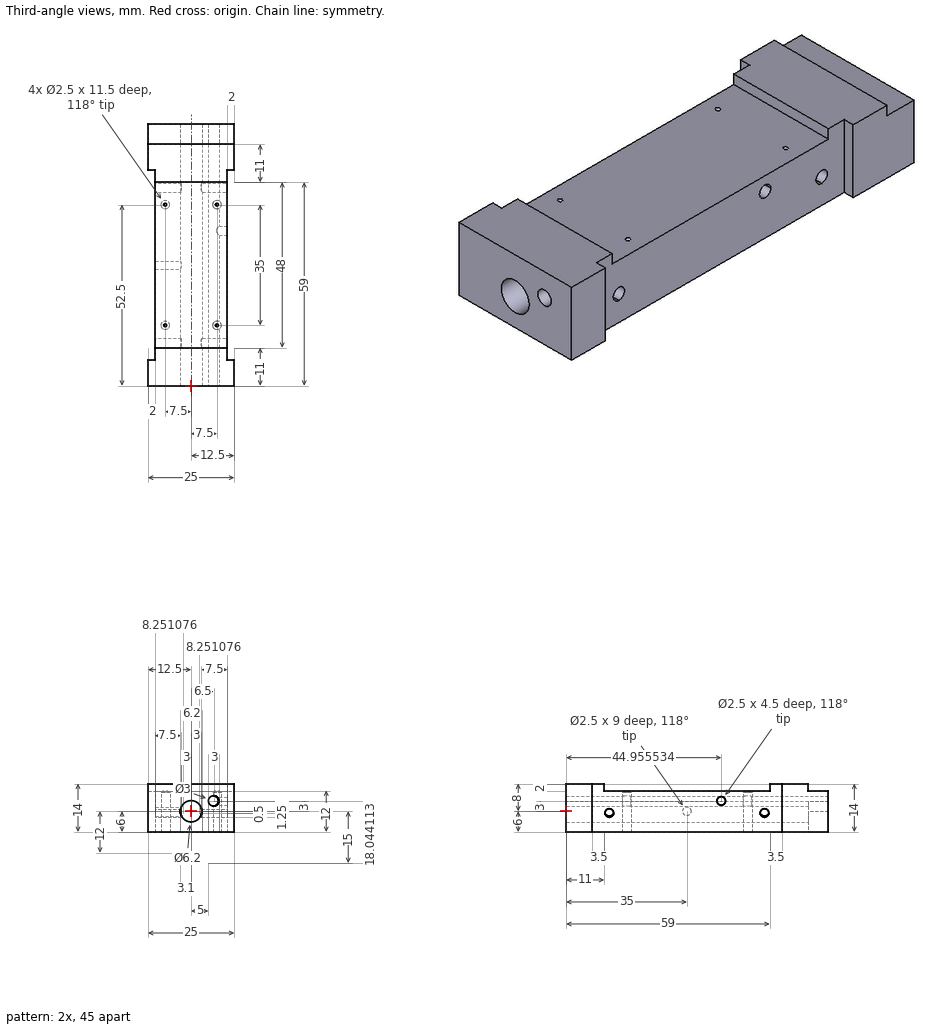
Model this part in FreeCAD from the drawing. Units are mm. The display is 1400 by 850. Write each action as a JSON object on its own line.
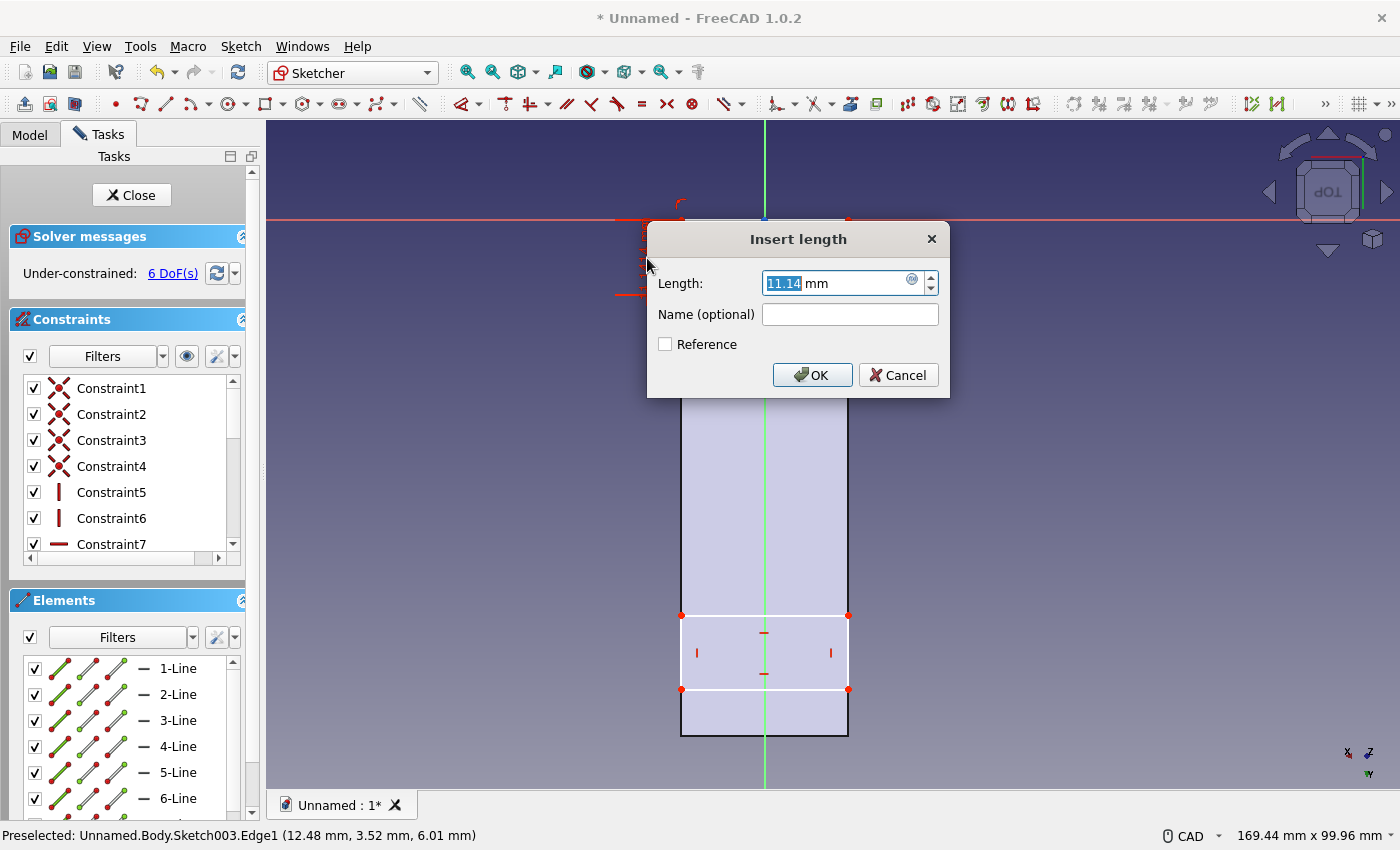
{"action": "type", "text": "11"}
{"action": "key", "text": "Return"}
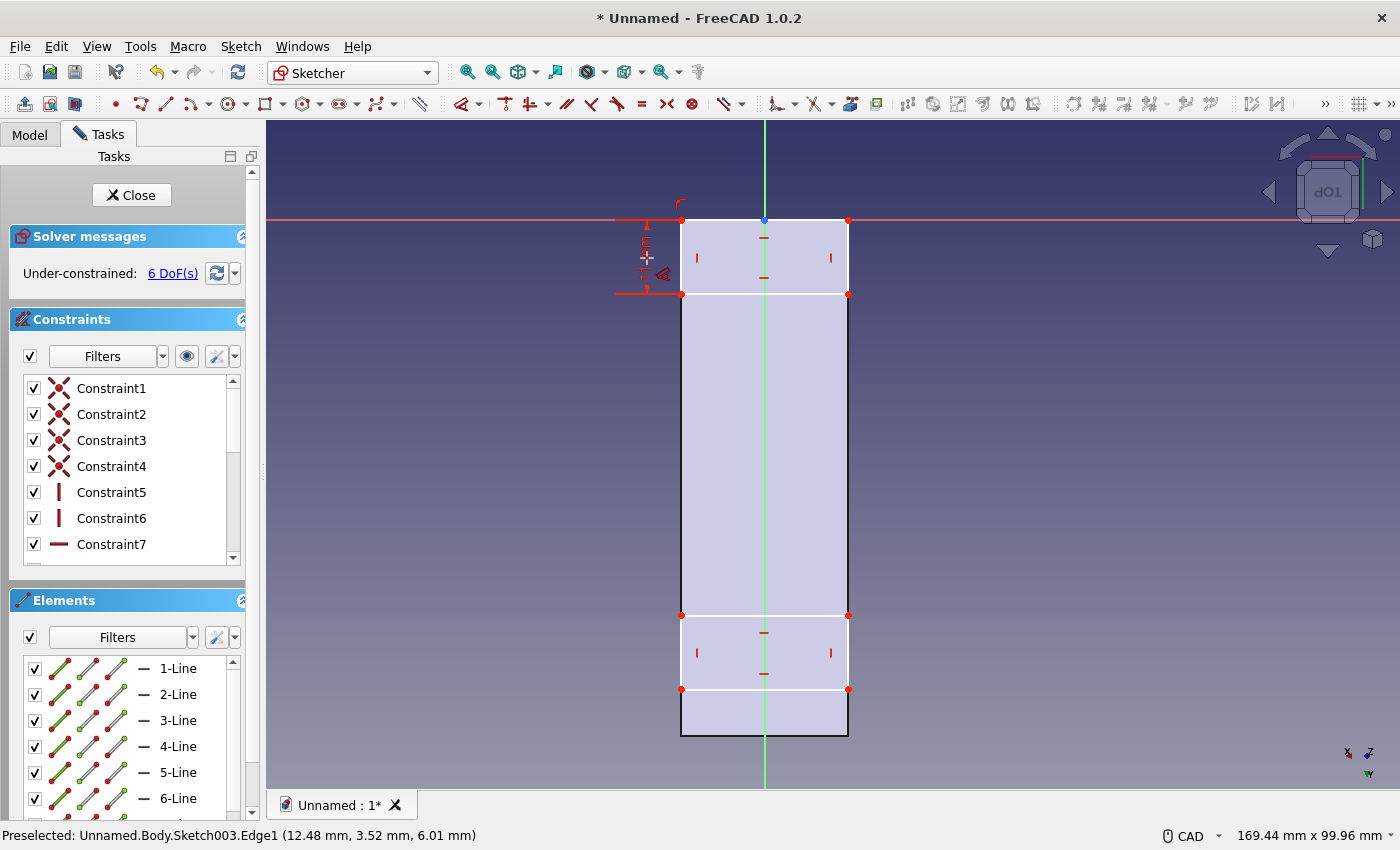
{"action": "left_click", "coordinate": [731, 294]}
{"action": "left_click", "coordinate": [726, 260]}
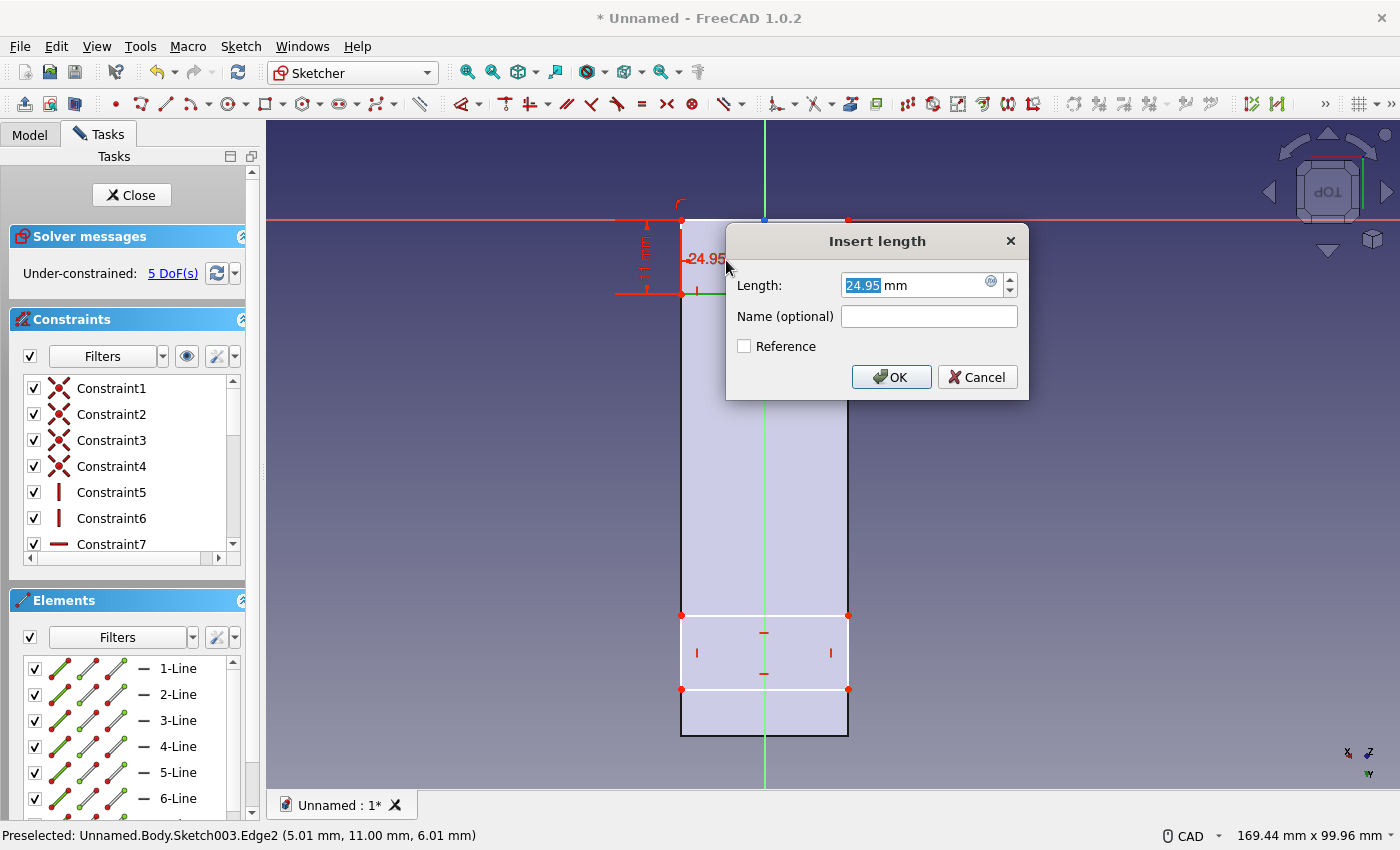
{"action": "type", "text": "25"}
{"action": "key", "text": "Return"}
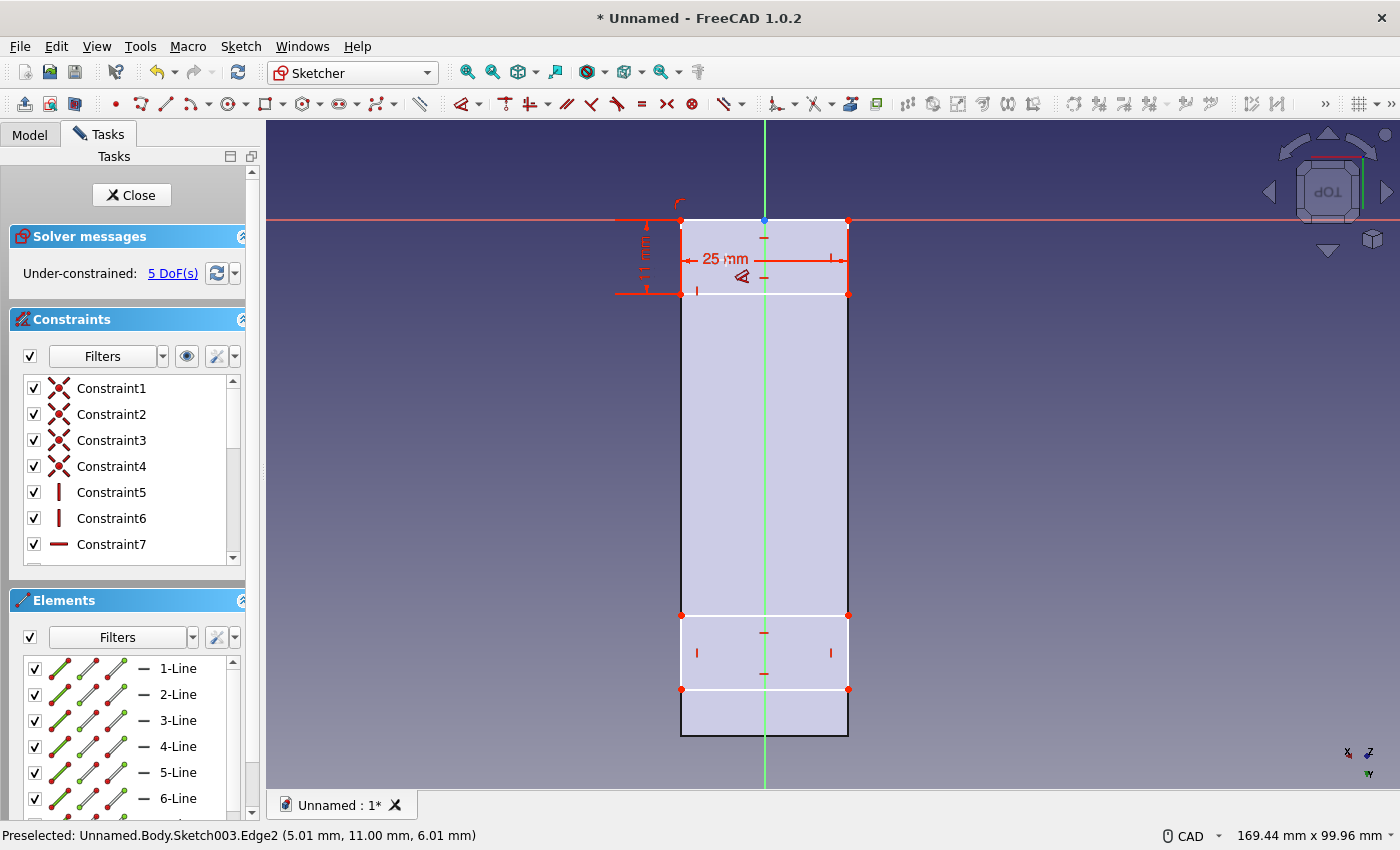
{"action": "left_click", "coordinate": [681, 638]}
{"action": "left_click", "coordinate": [647, 653]}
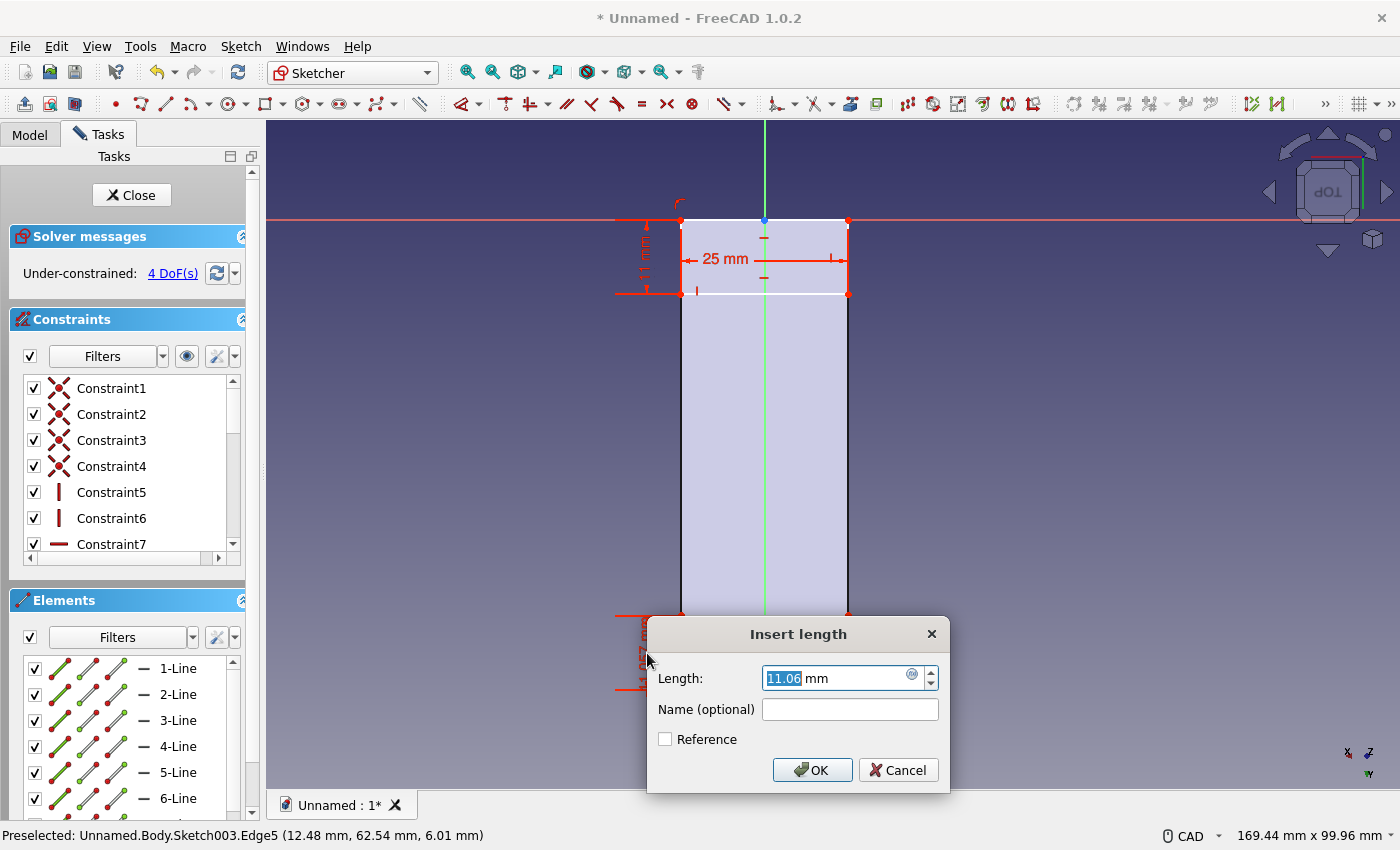
{"action": "type", "text": "11"}
{"action": "key", "text": "Return"}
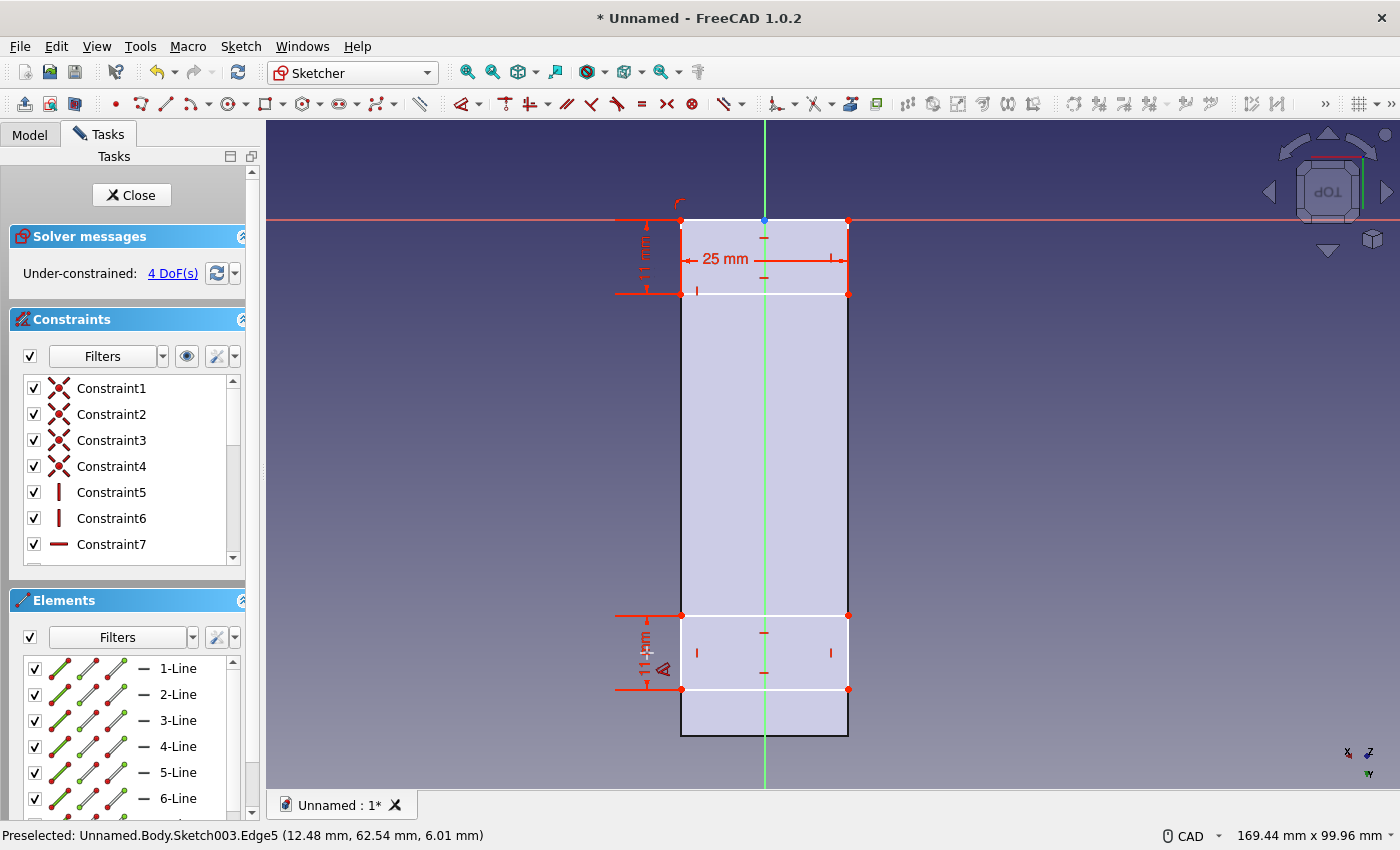
{"action": "left_click", "coordinate": [731, 690]}
{"action": "left_click", "coordinate": [726, 724]}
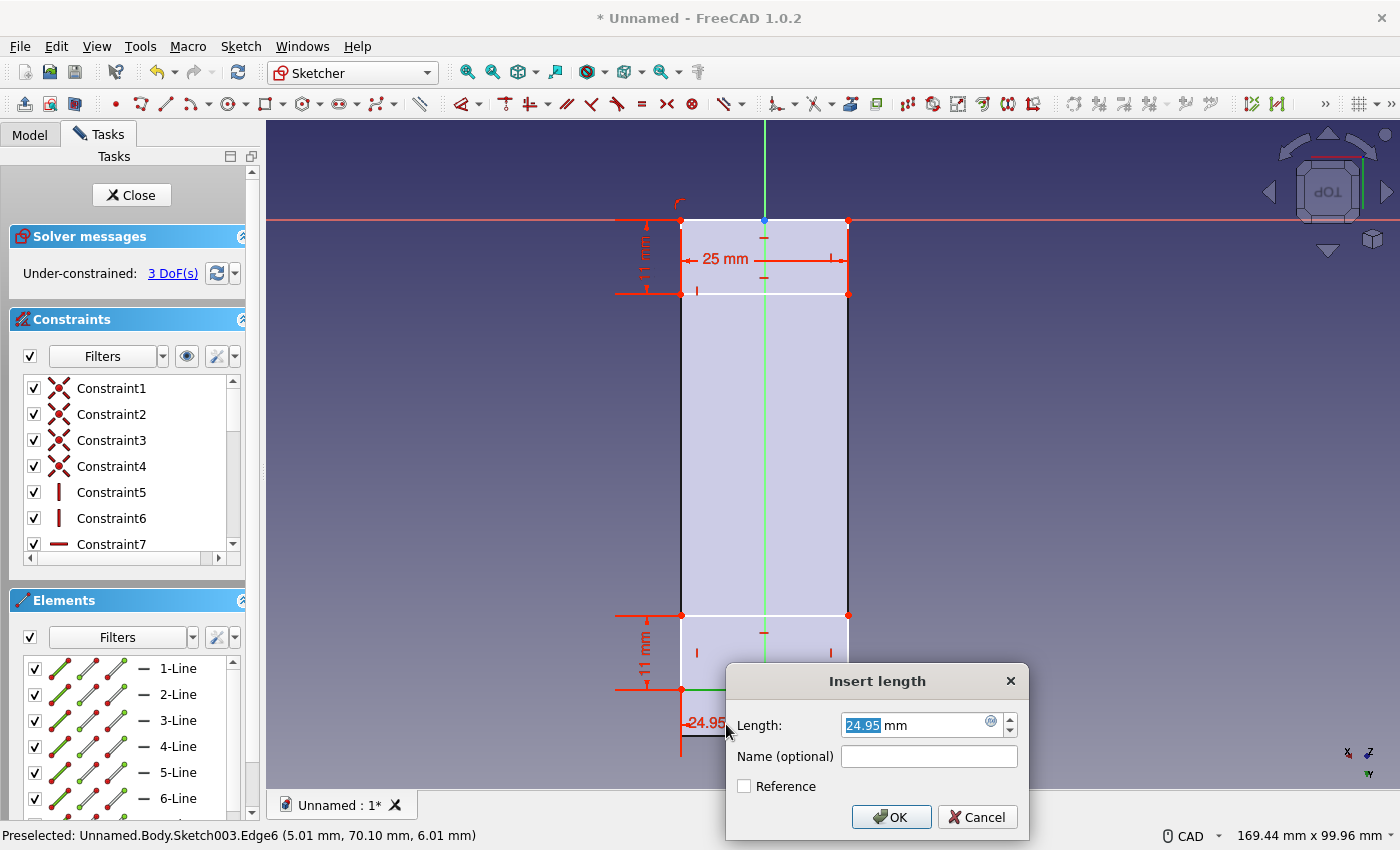
{"action": "type", "text": "25"}
{"action": "key", "text": "Return"}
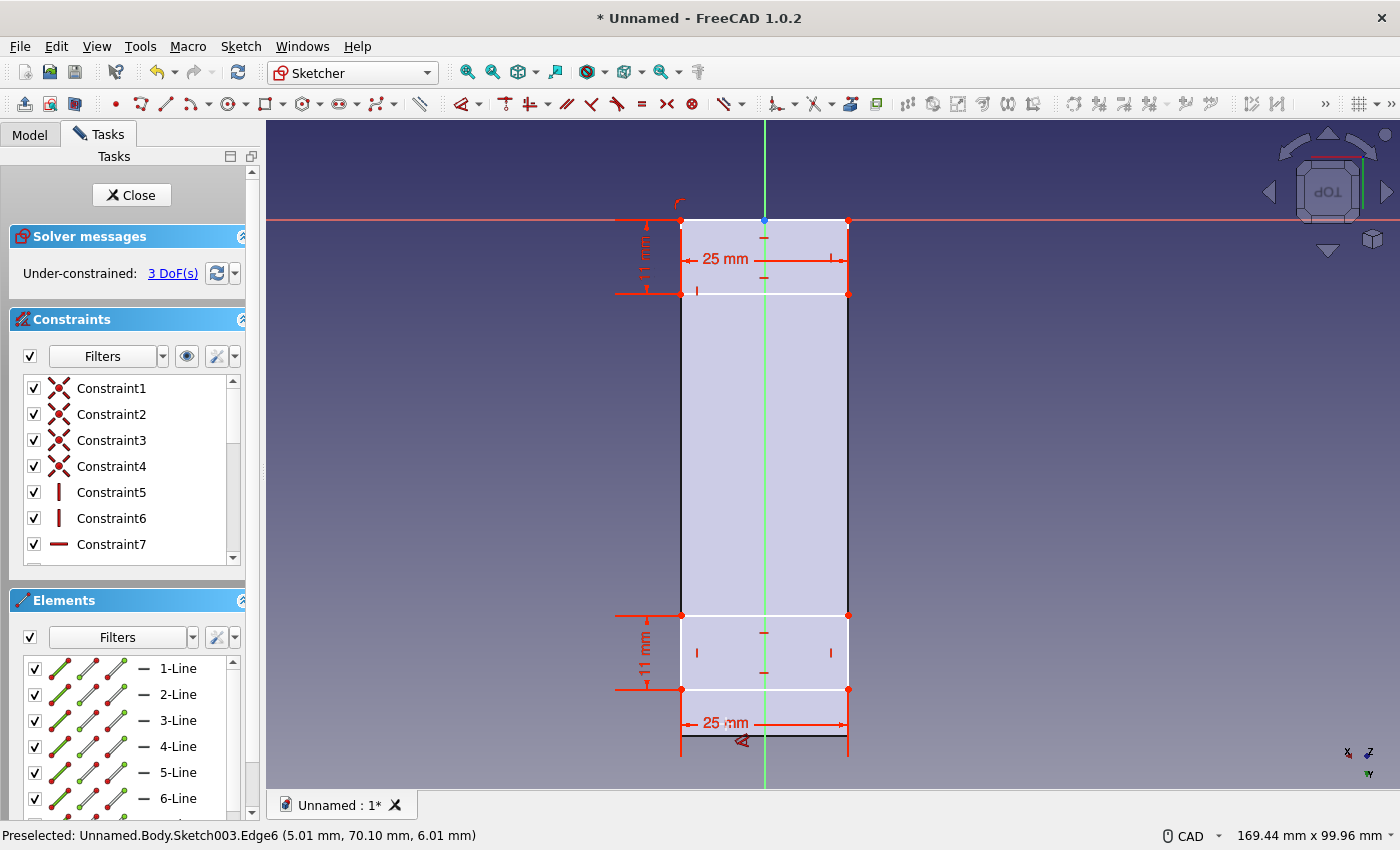
{"action": "left_click", "coordinate": [681, 616]}
{"action": "left_click", "coordinate": [647, 418]}